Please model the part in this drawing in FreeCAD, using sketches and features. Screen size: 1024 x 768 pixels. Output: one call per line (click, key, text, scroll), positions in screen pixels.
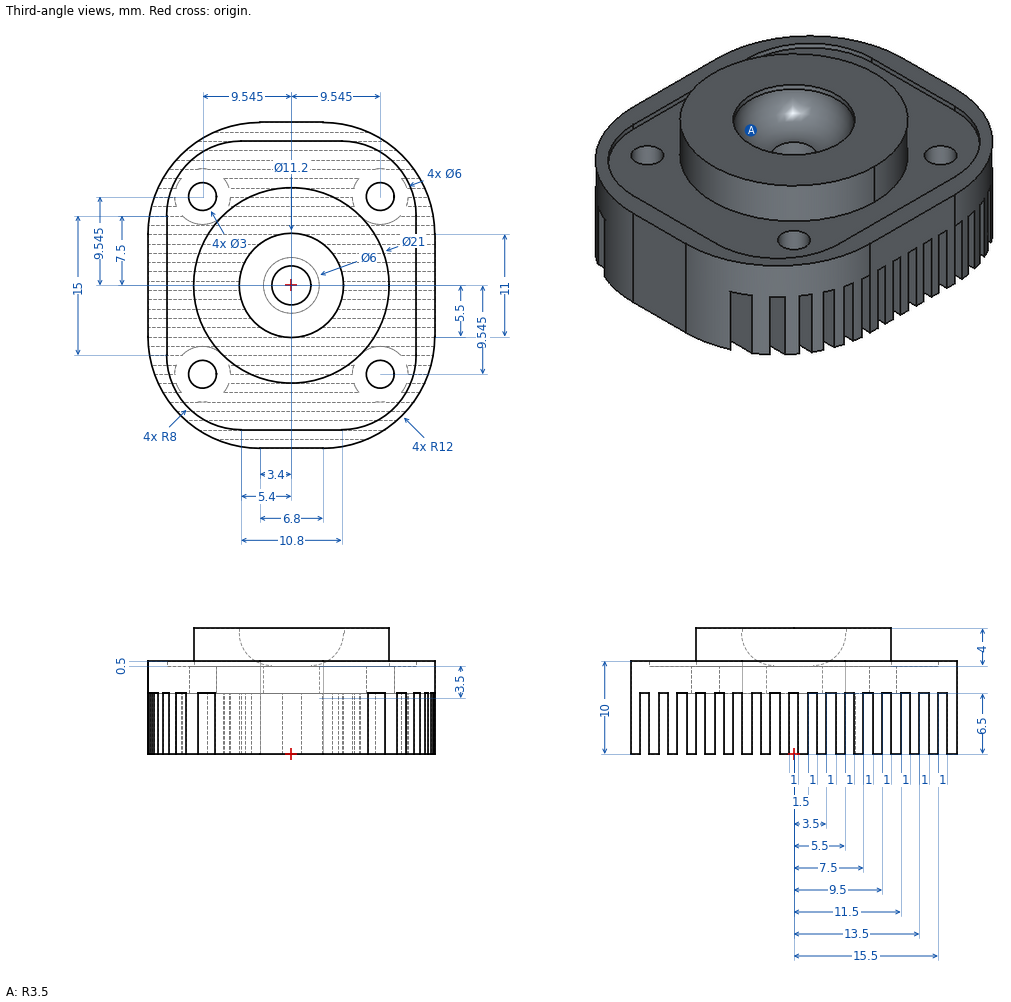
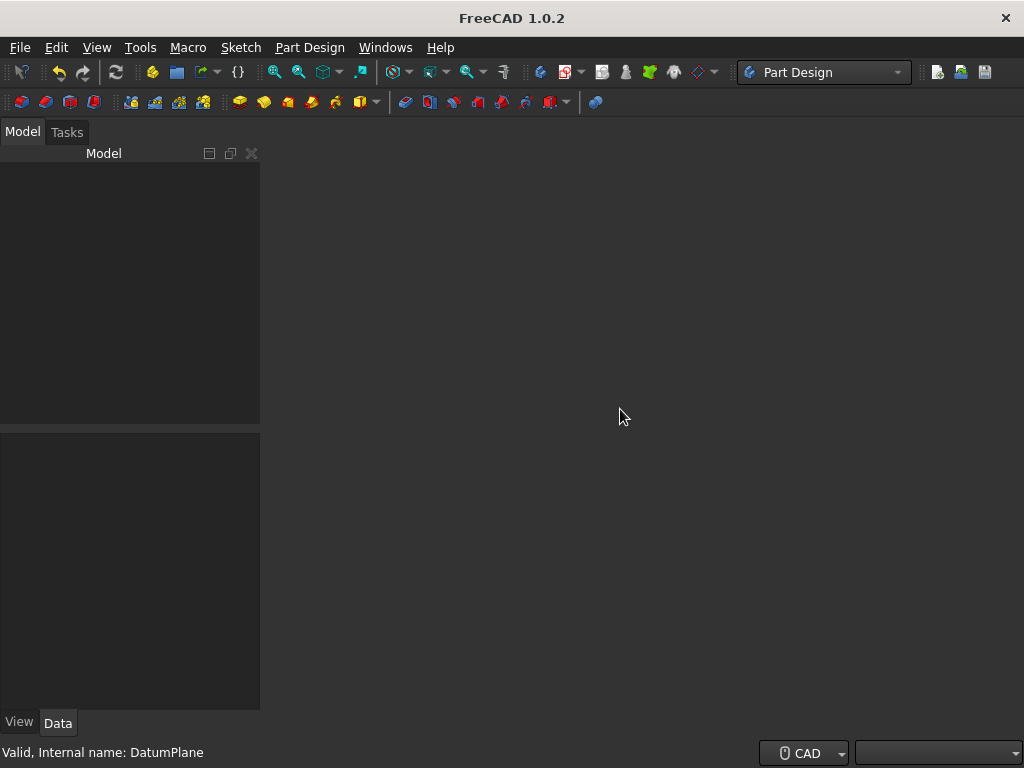
click(938, 72)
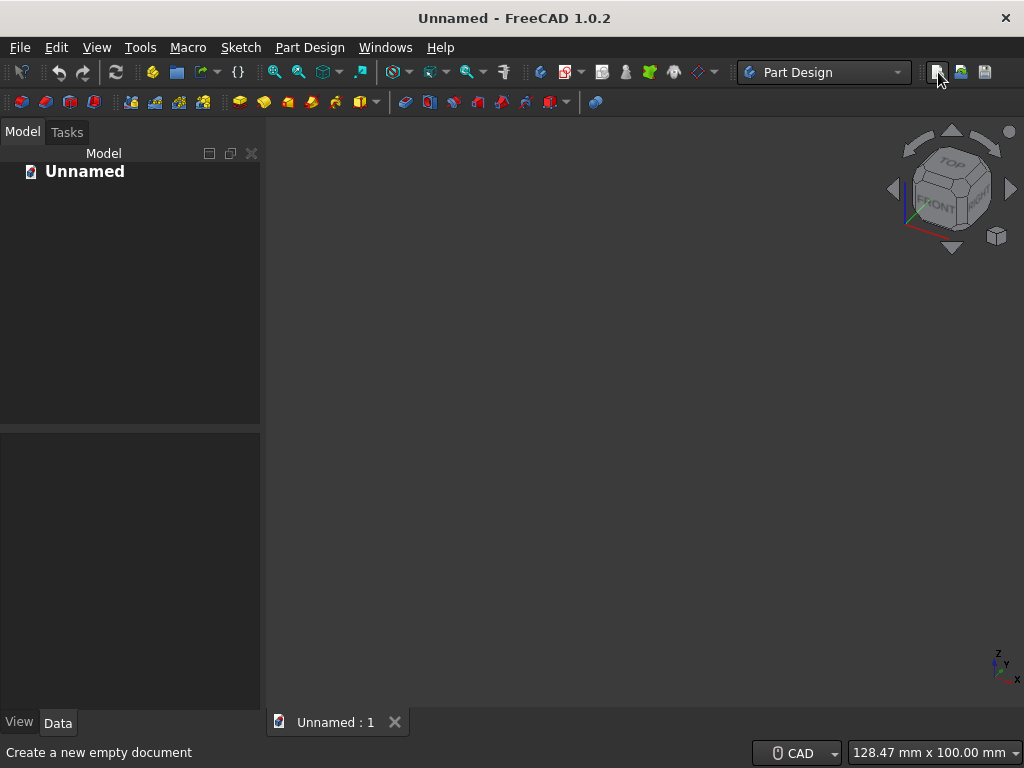
click(566, 72)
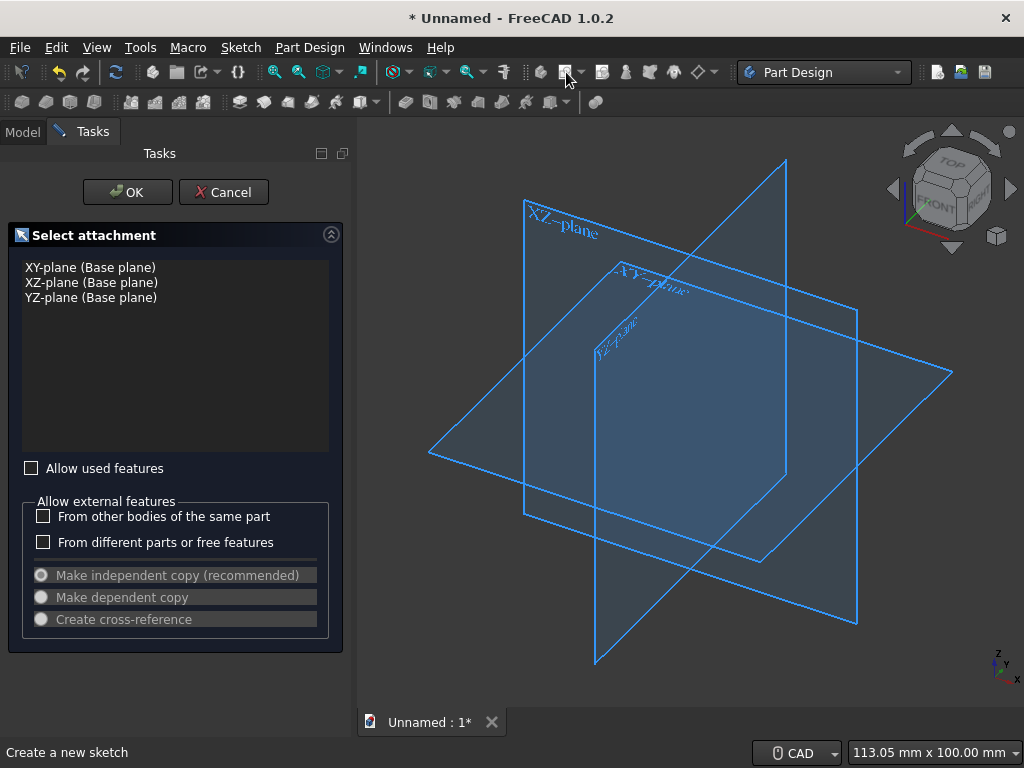
click(82, 268)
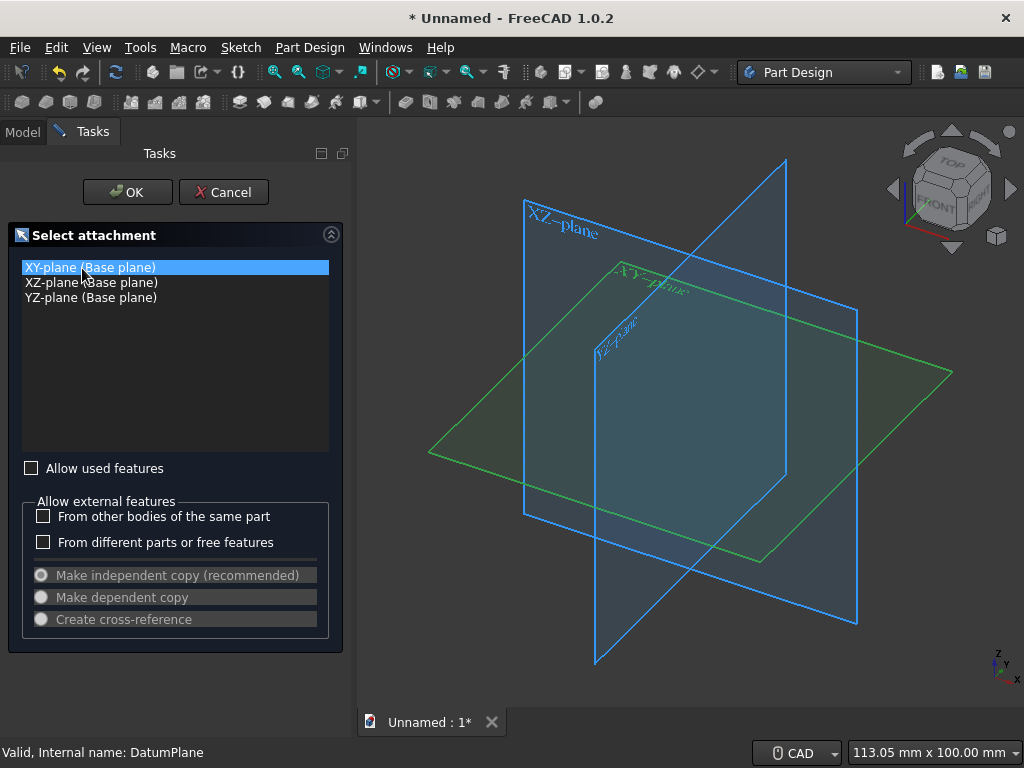
click(128, 192)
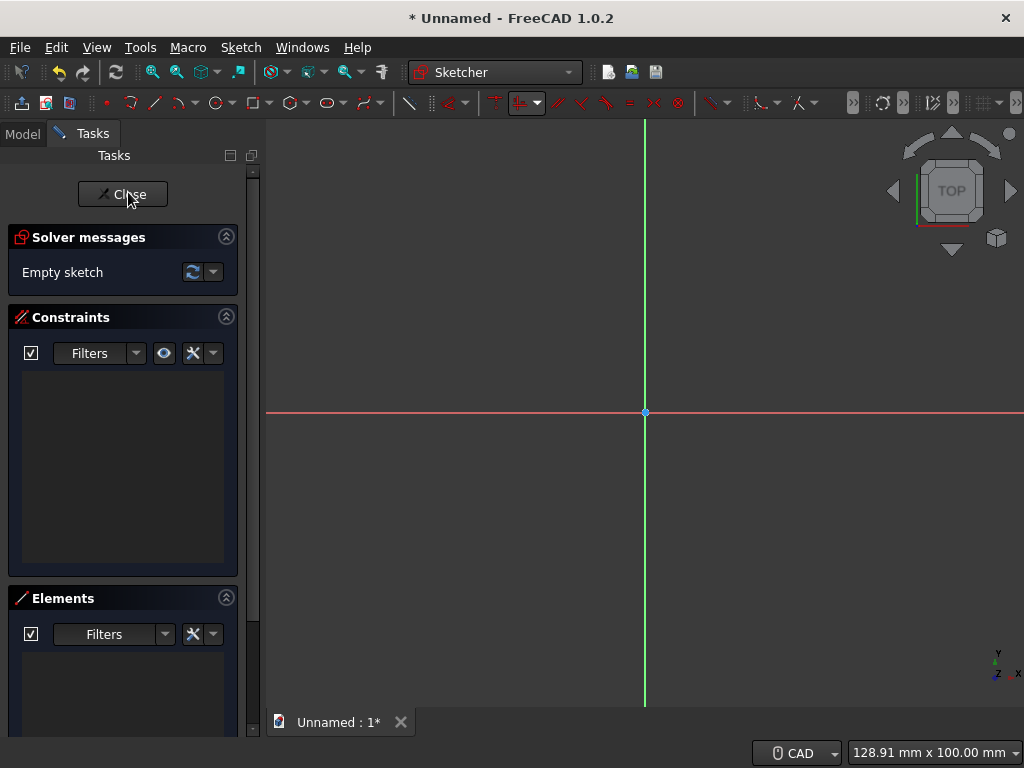
scroll(728, 413, up, 3)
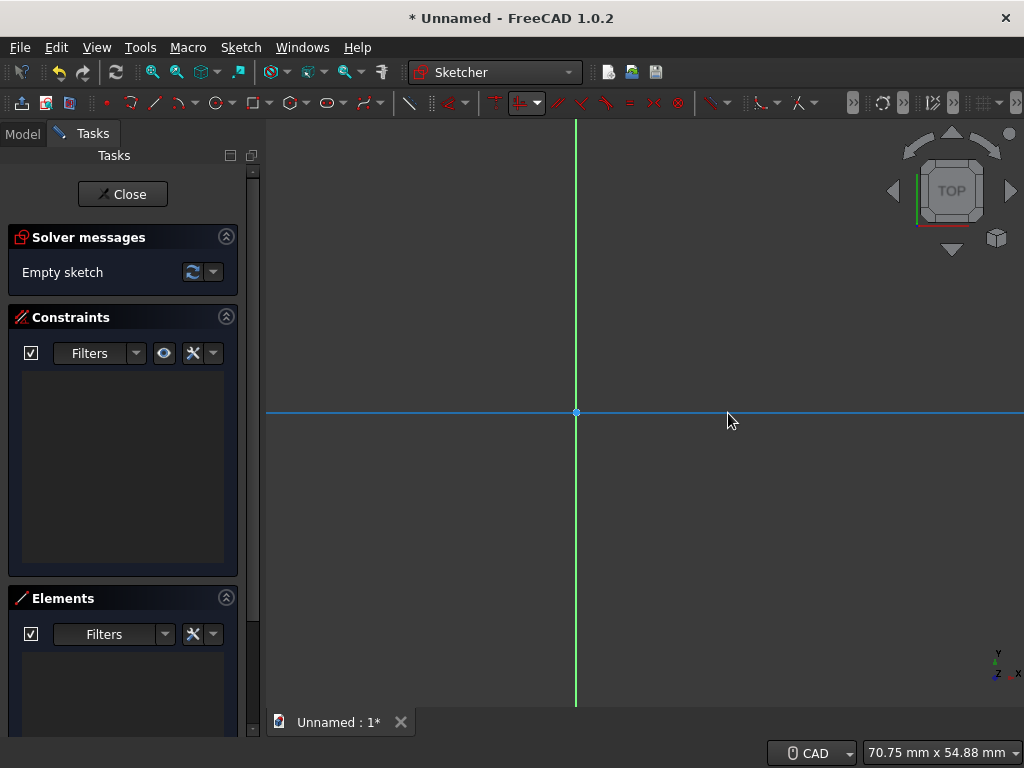
click(156, 104)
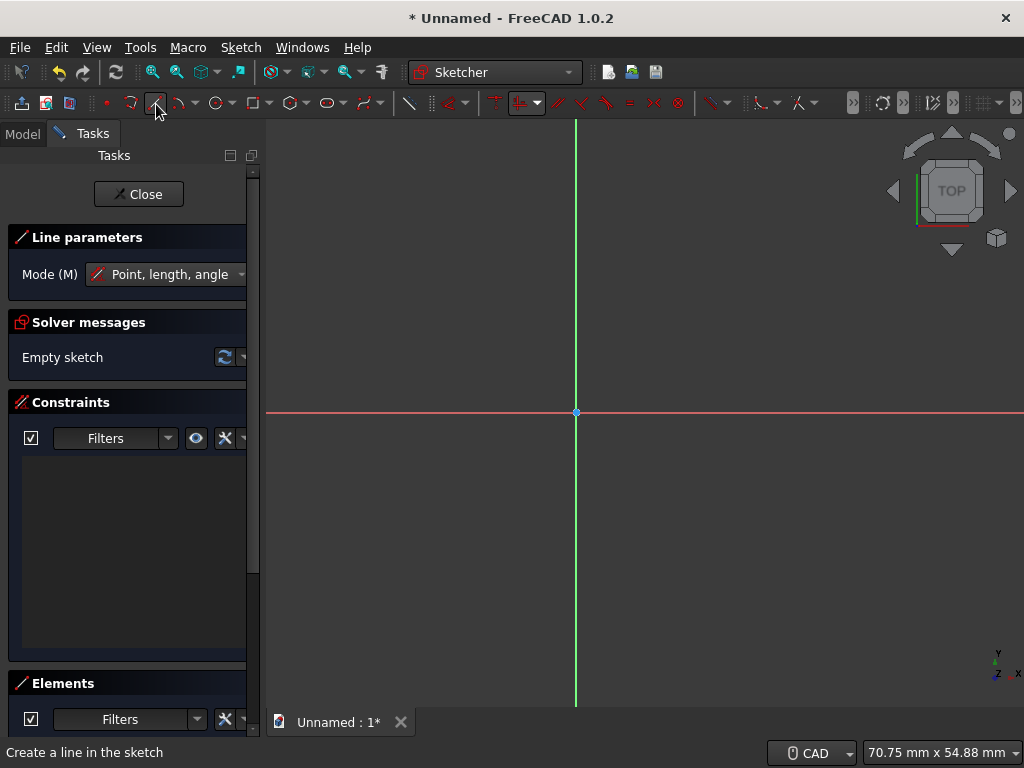
click(540, 600)
click(613, 600)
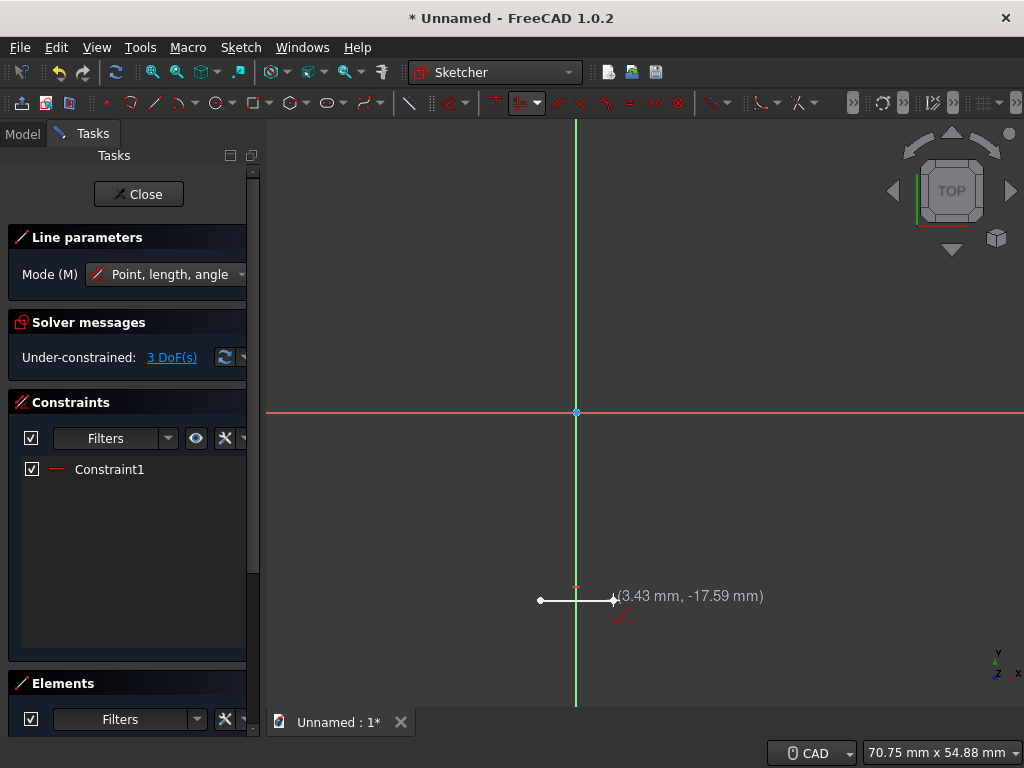
click(741, 472)
click(741, 354)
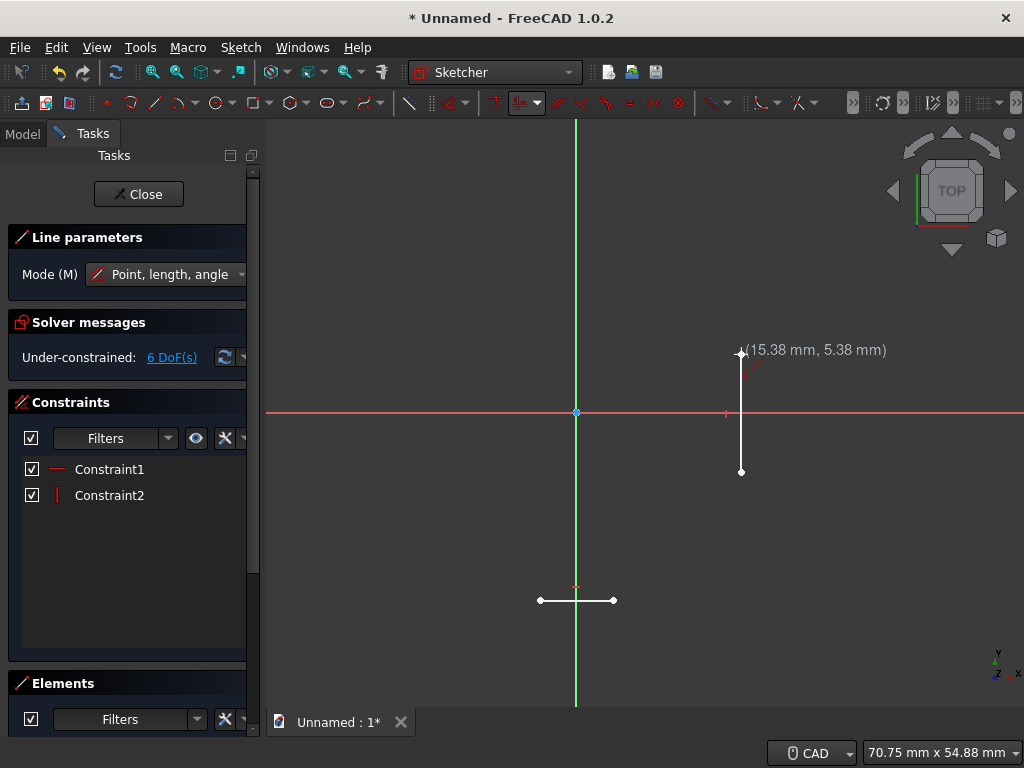
click(613, 225)
click(540, 225)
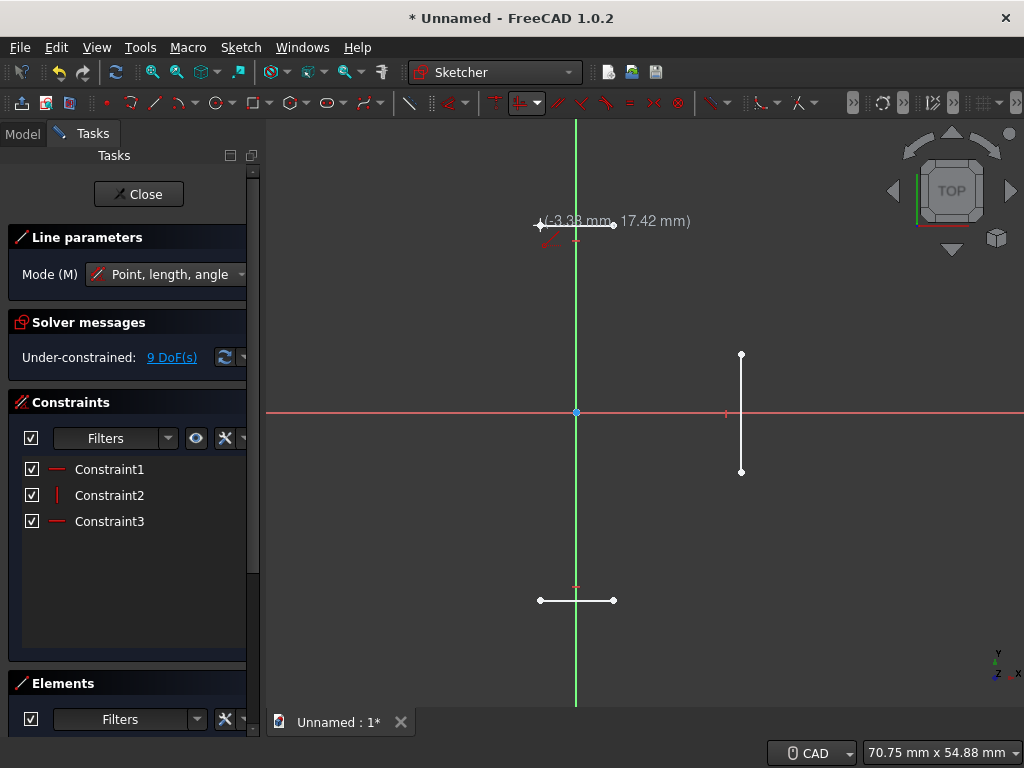
click(411, 354)
click(411, 472)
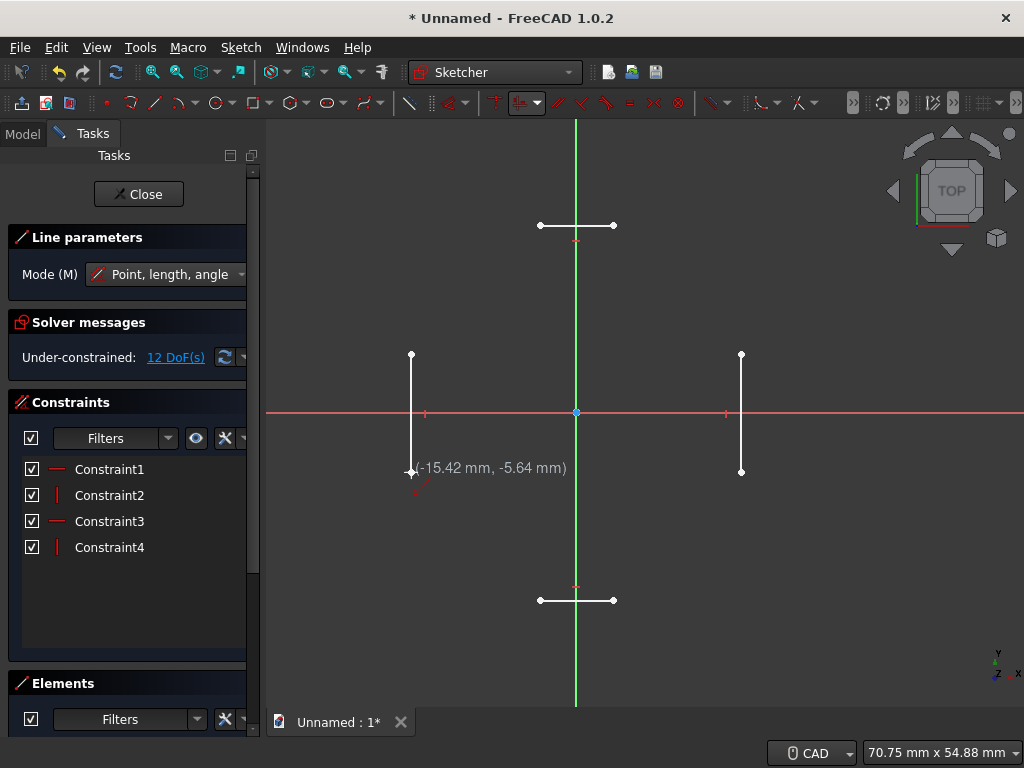
key(g)
key(3)
key(a)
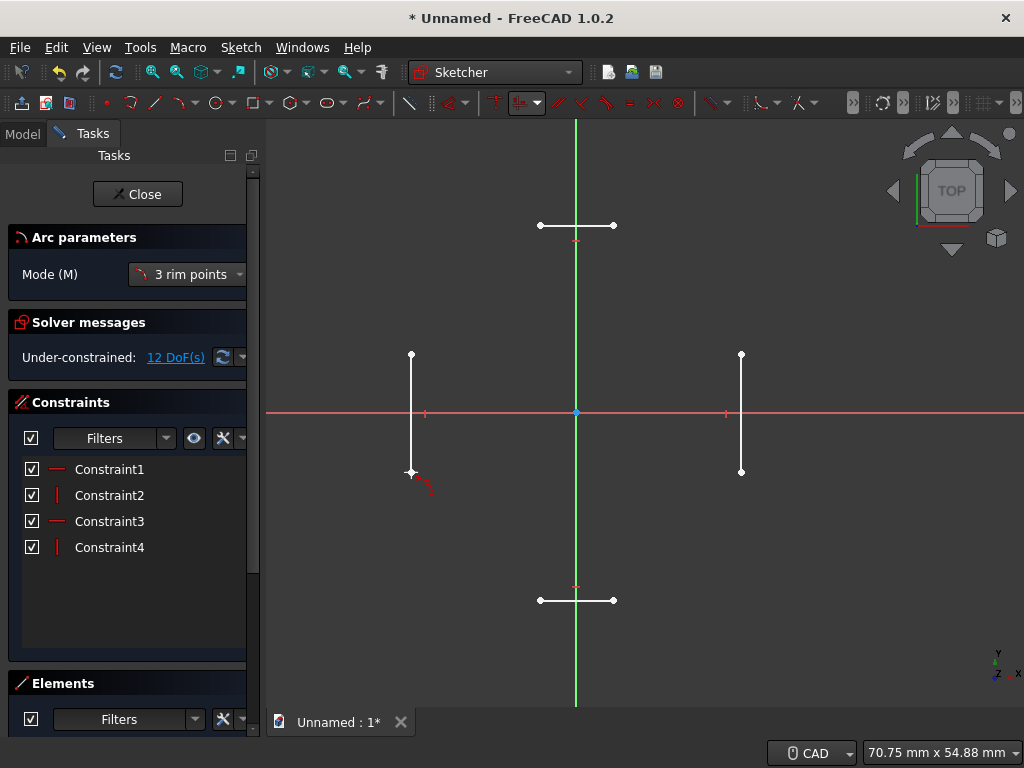
click(613, 601)
click(741, 473)
click(704, 562)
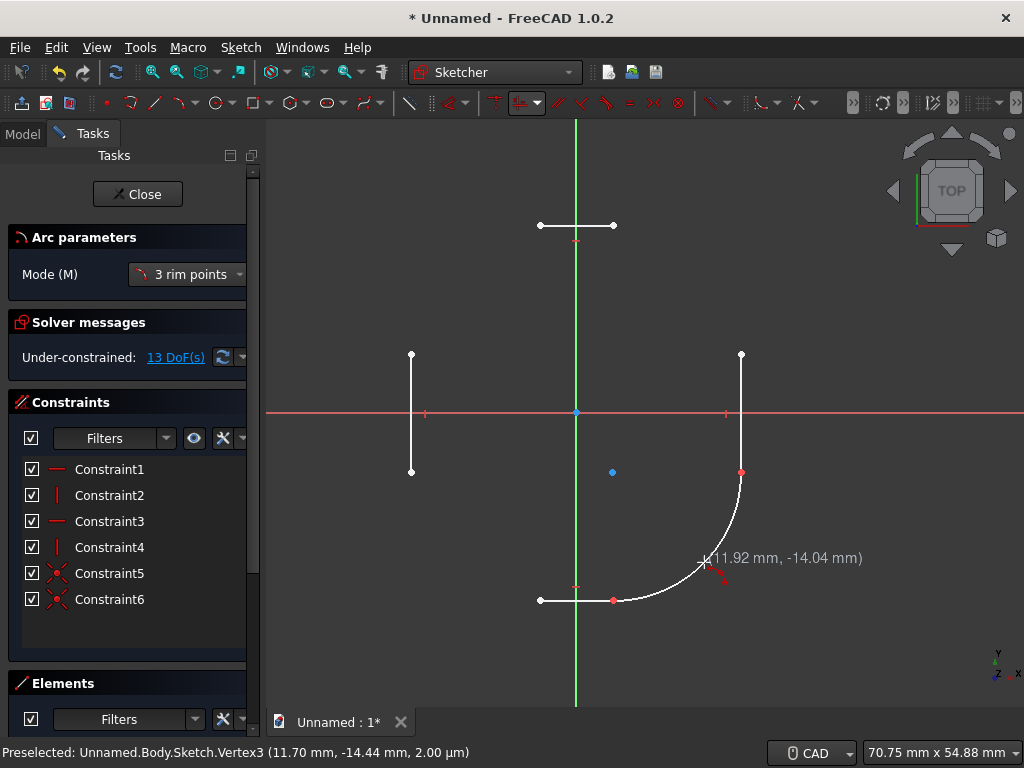
click(741, 355)
click(613, 226)
click(704, 263)